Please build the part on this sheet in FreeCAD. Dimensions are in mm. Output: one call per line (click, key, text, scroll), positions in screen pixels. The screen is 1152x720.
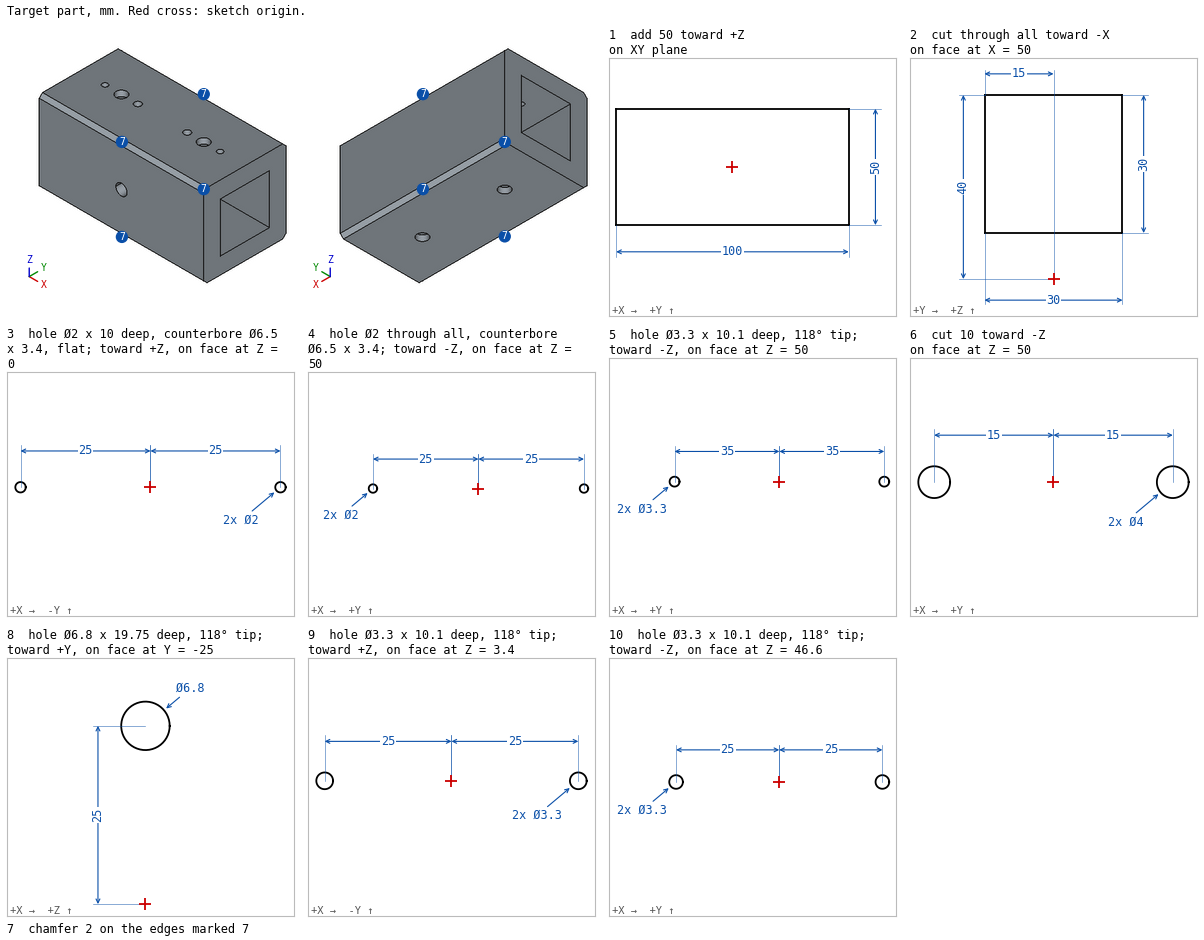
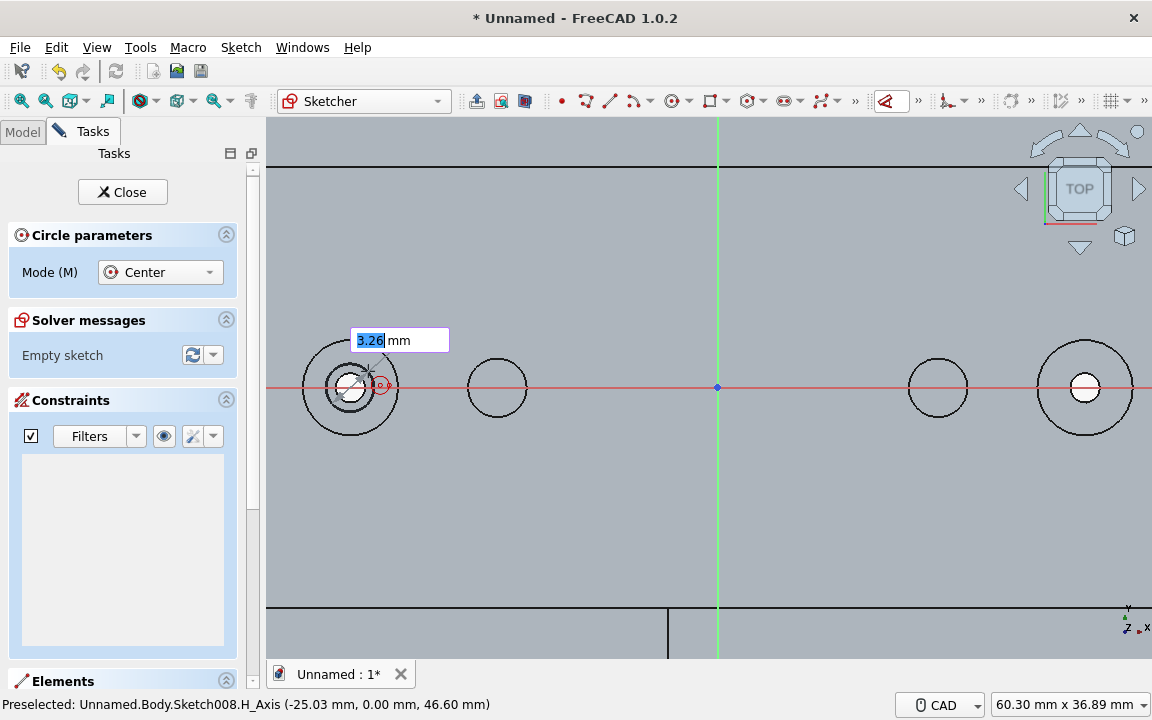
text(3.3)
key(Return)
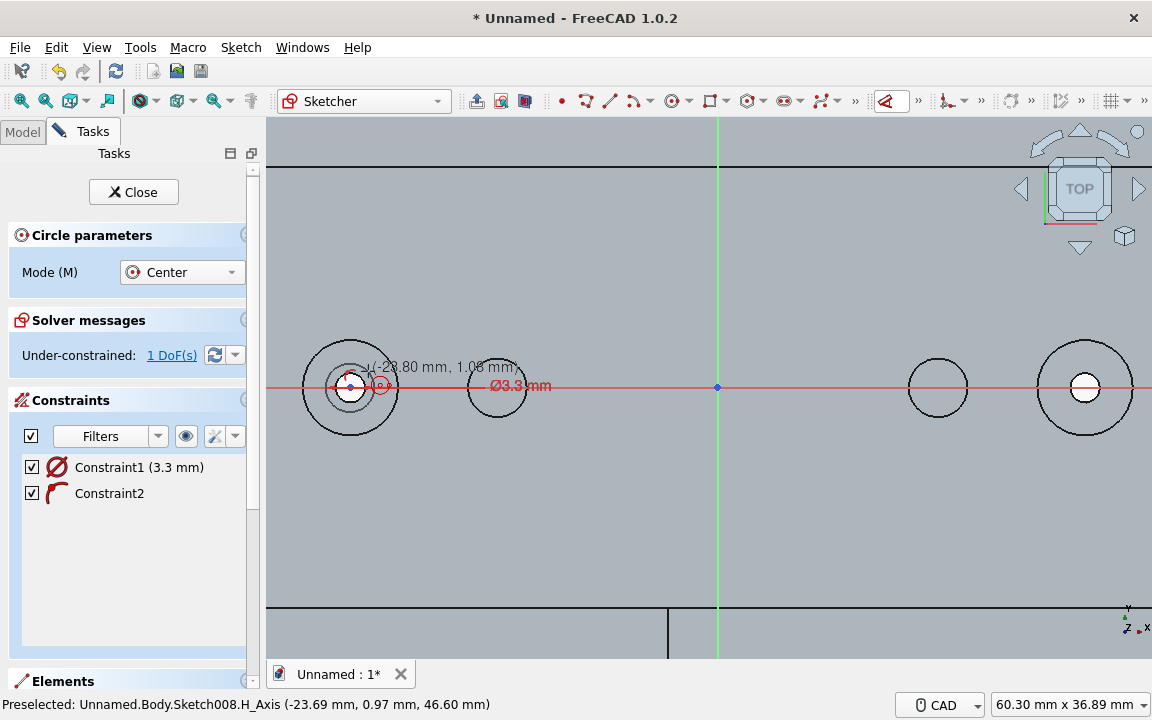
scroll(483, 388, down, 2)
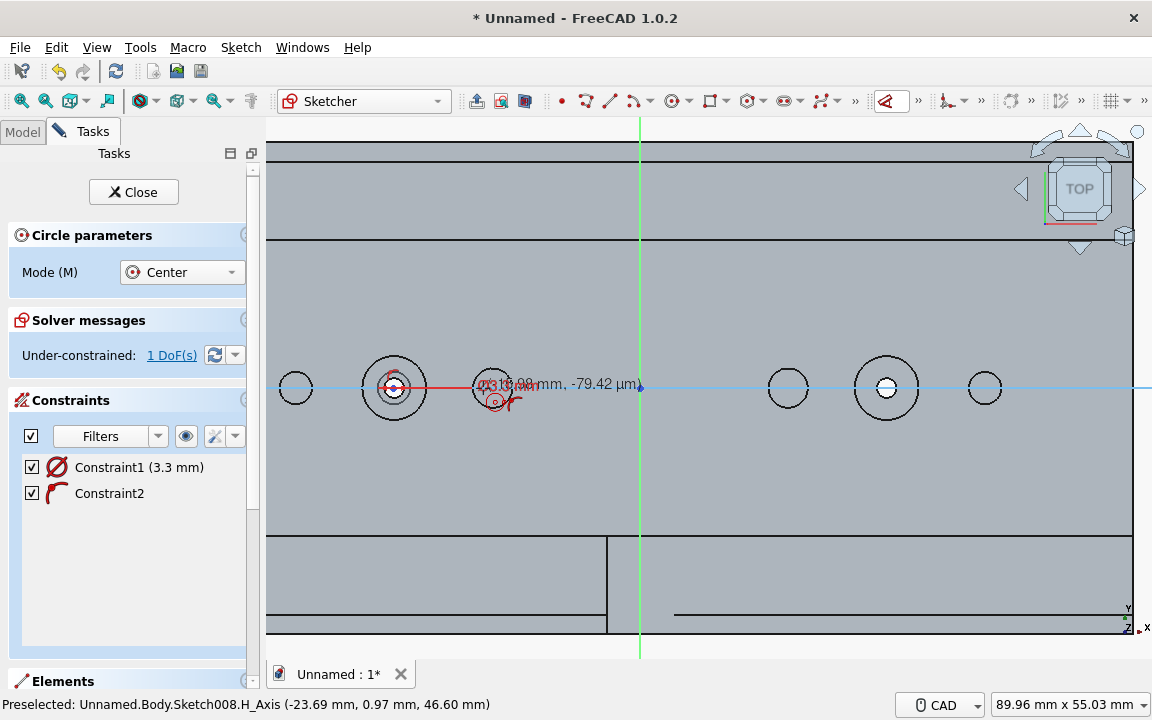
scroll(887, 388, up, 2)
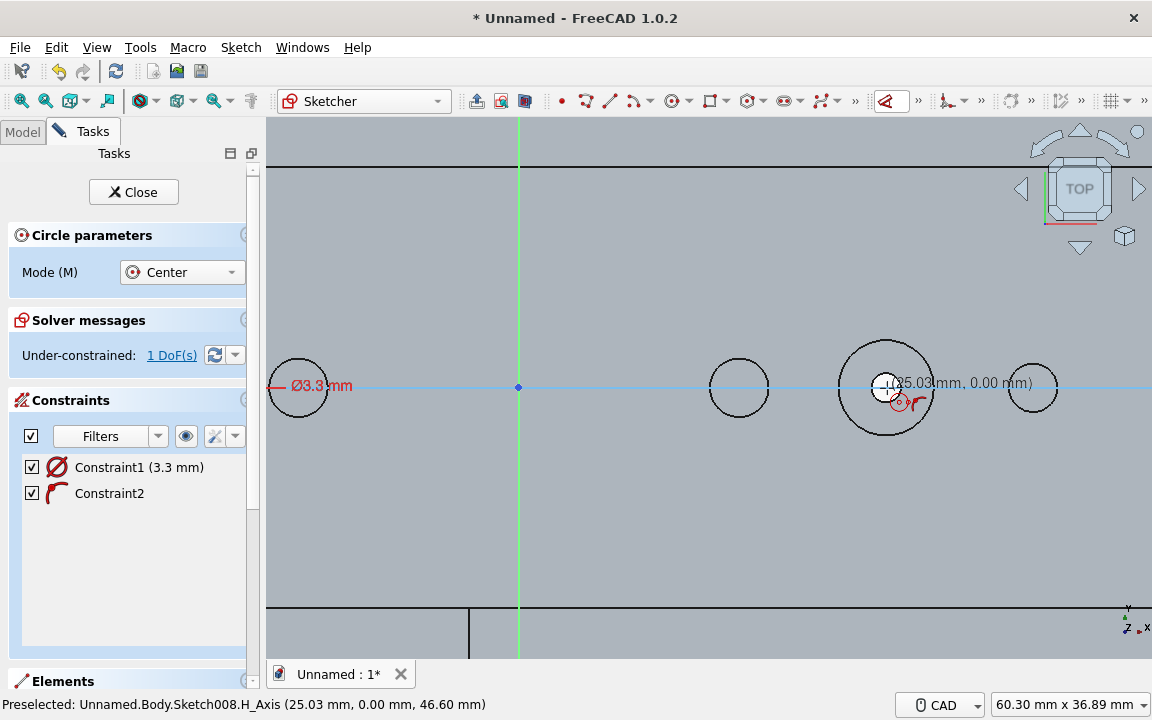
click(886, 388)
move(903, 371)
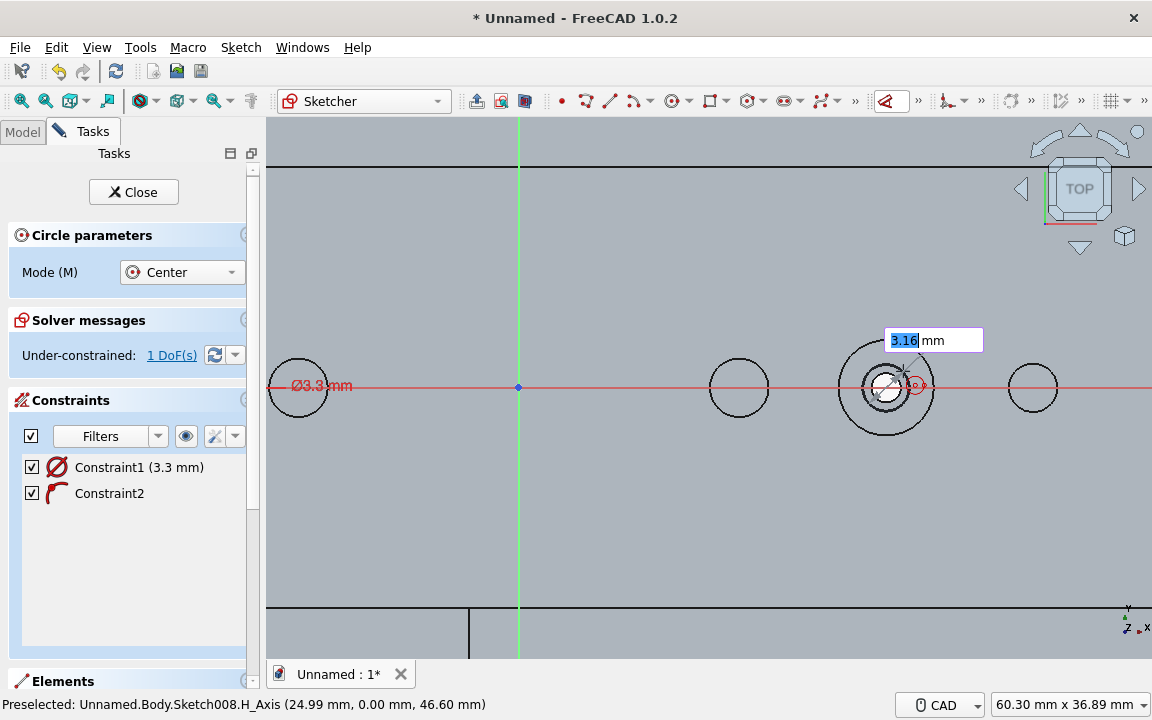
text(3.3)
key(Return)
key(Escape)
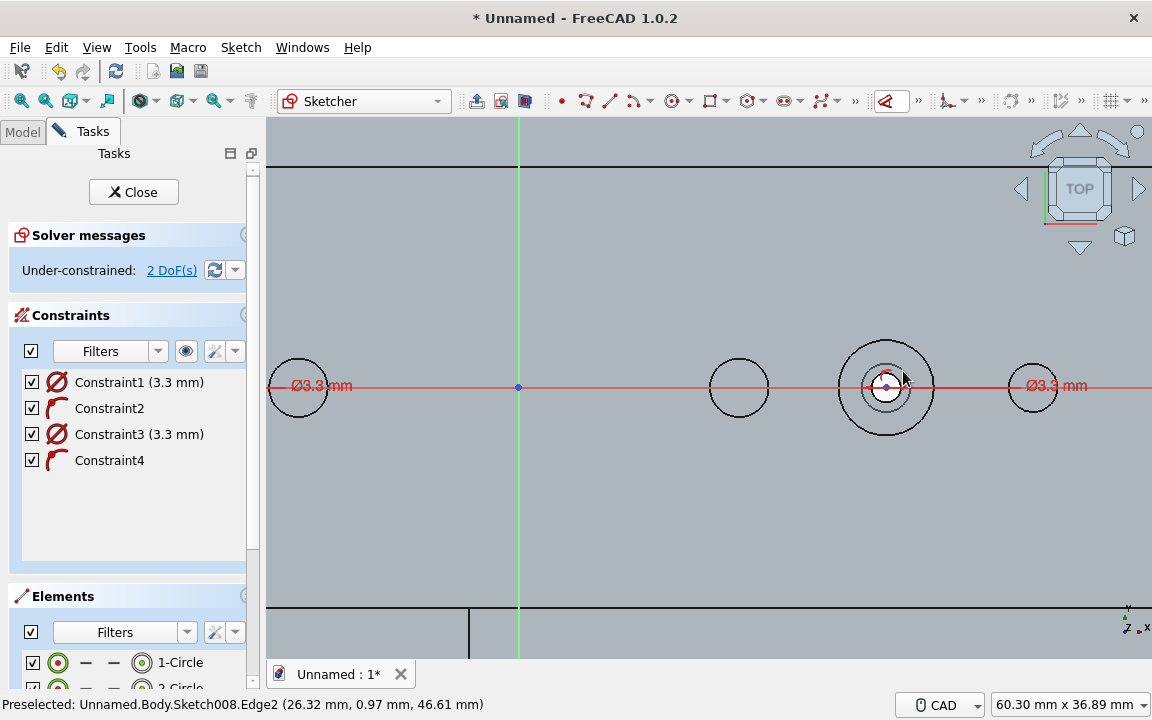
scroll(888, 388, down, 2)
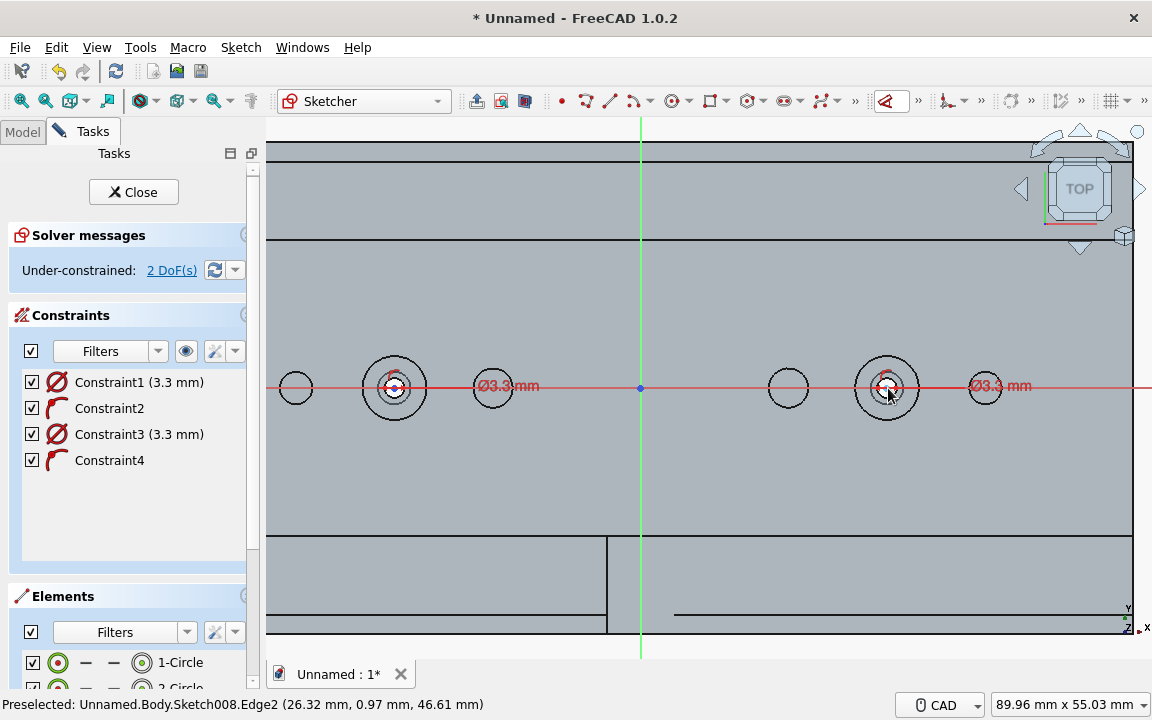
click(394, 388)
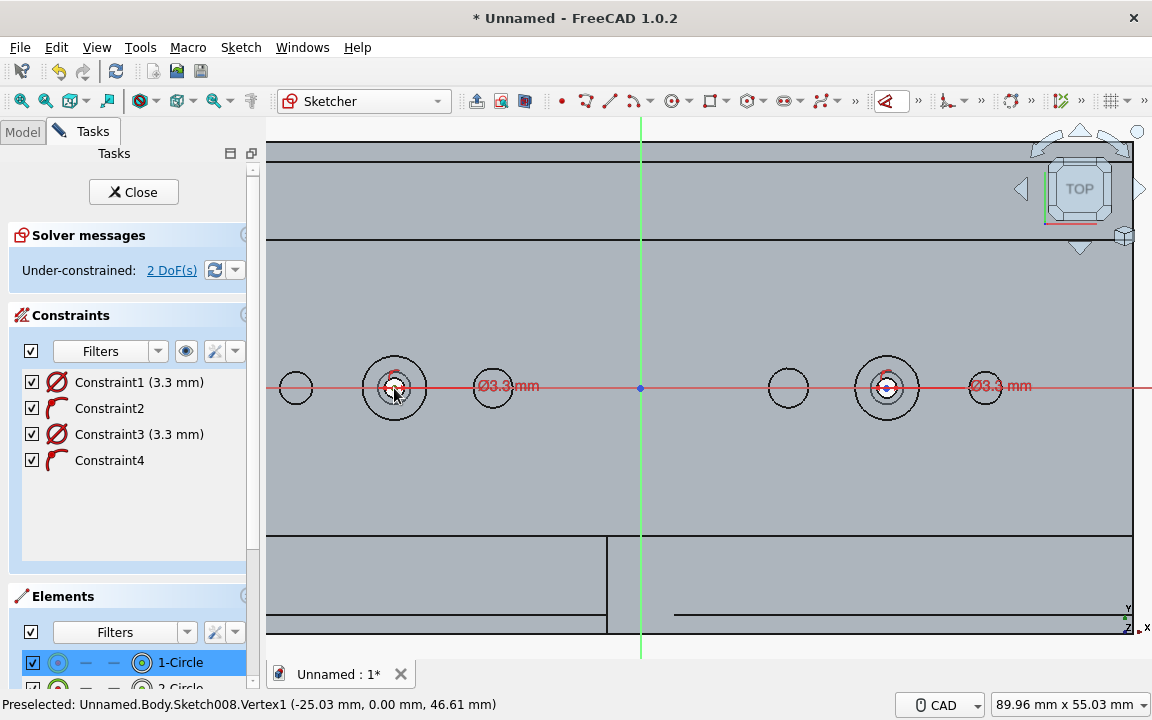
click(904, 102)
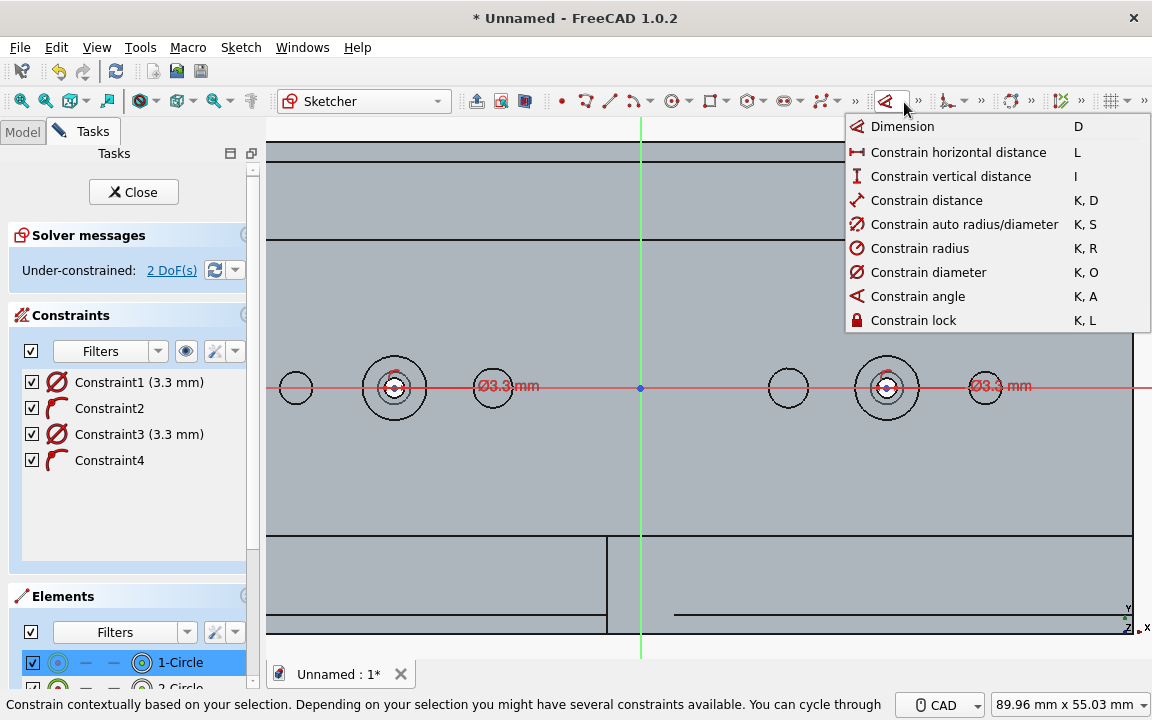
click(998, 152)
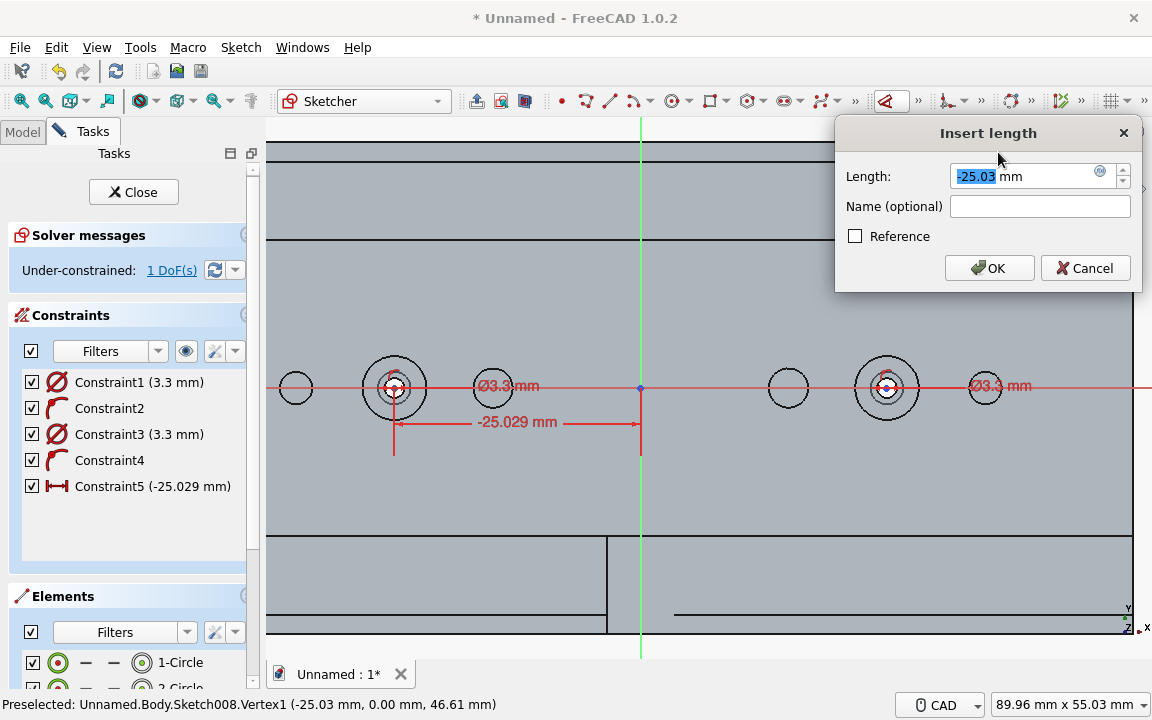
text(-25)
key(Return)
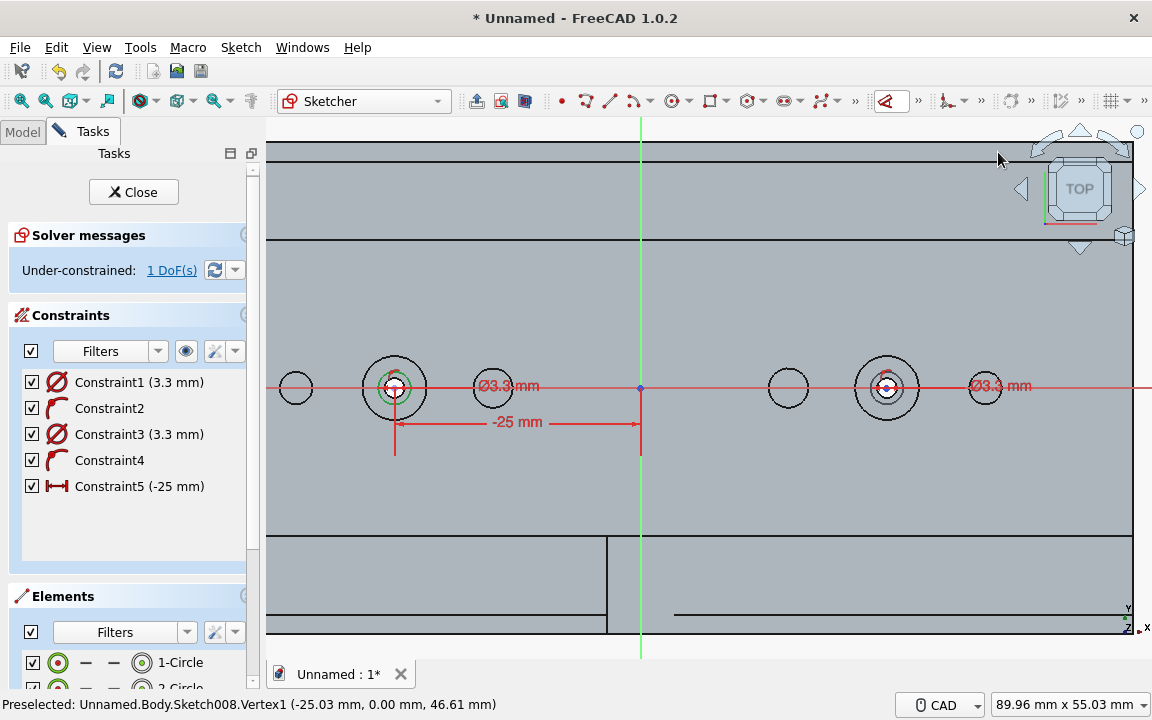
click(887, 388)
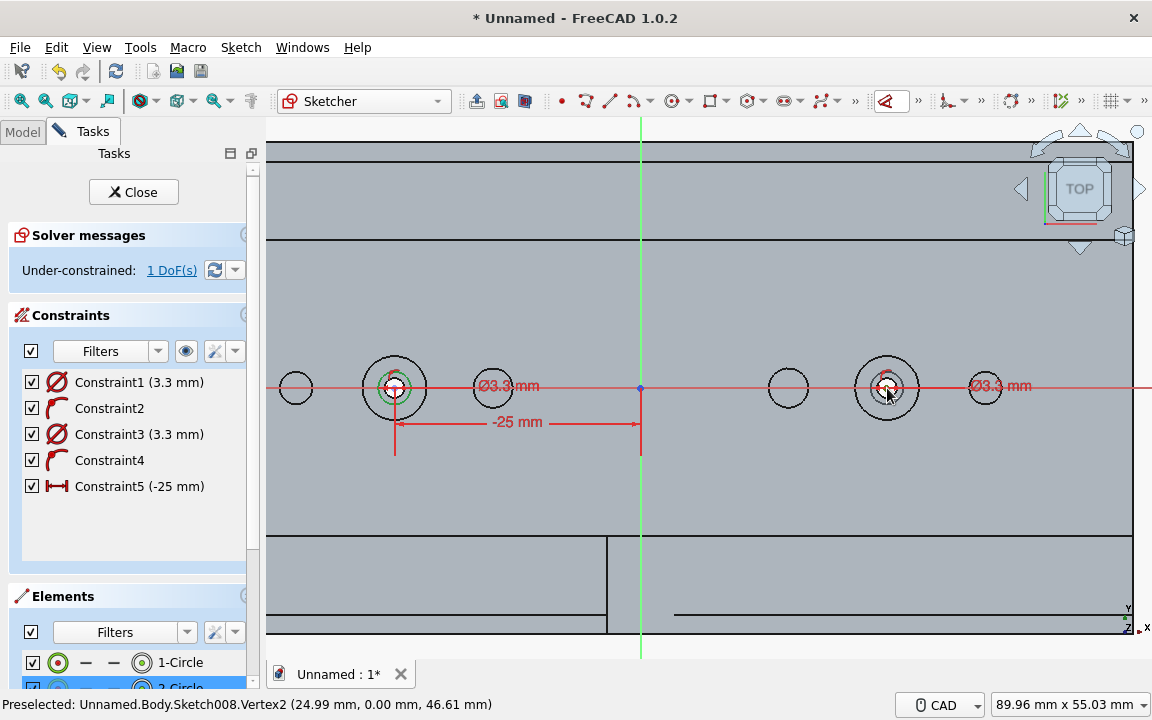
key(l)